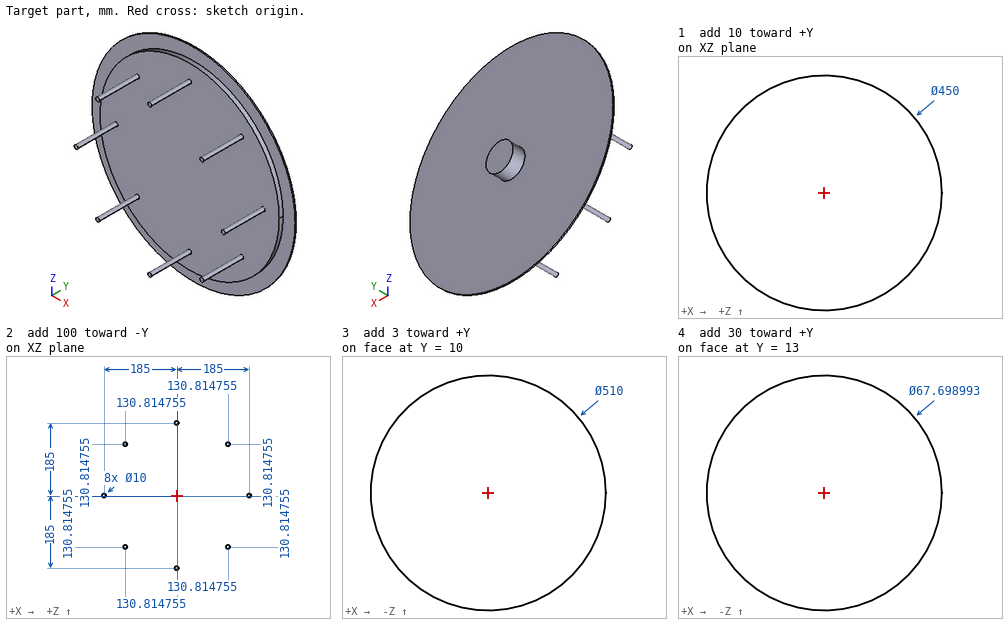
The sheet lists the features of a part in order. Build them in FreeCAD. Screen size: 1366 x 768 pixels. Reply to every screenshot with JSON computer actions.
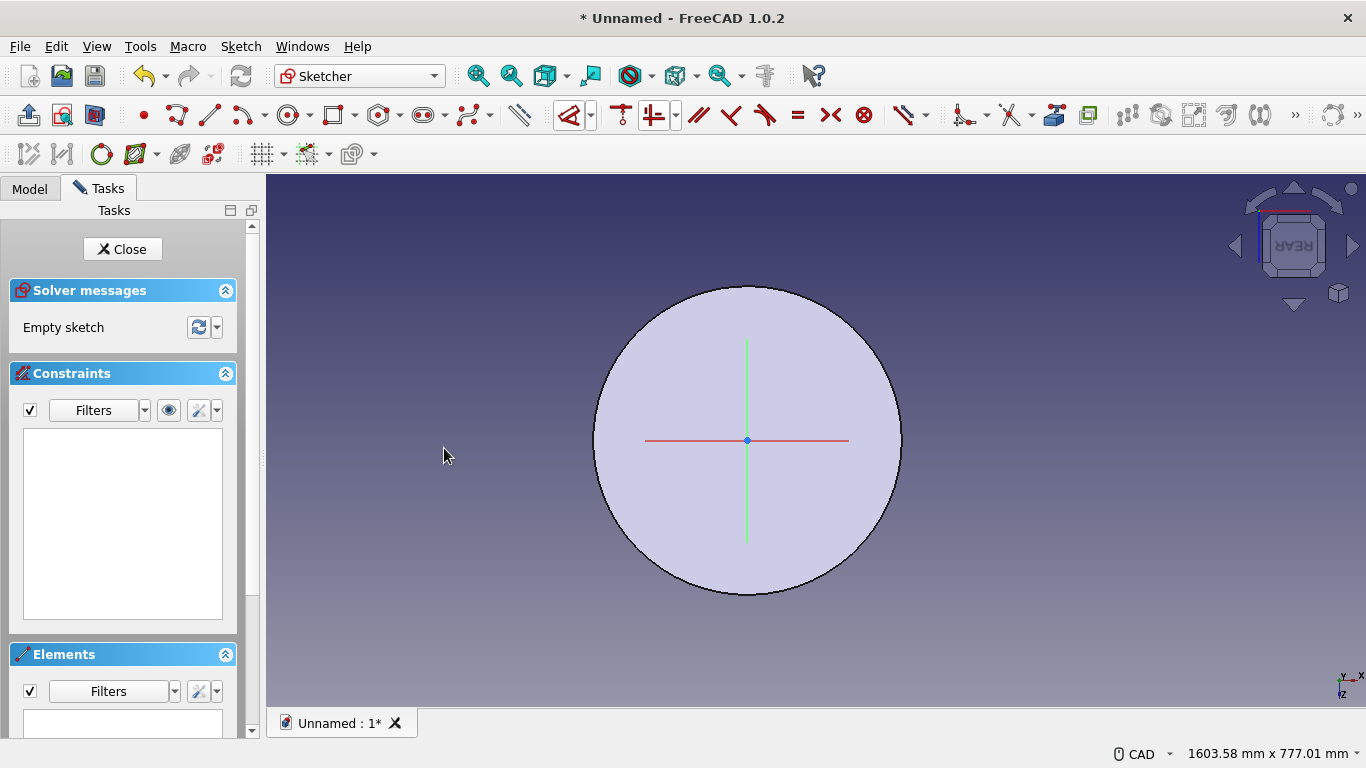
{"action": "left_click", "coordinate": [288, 116]}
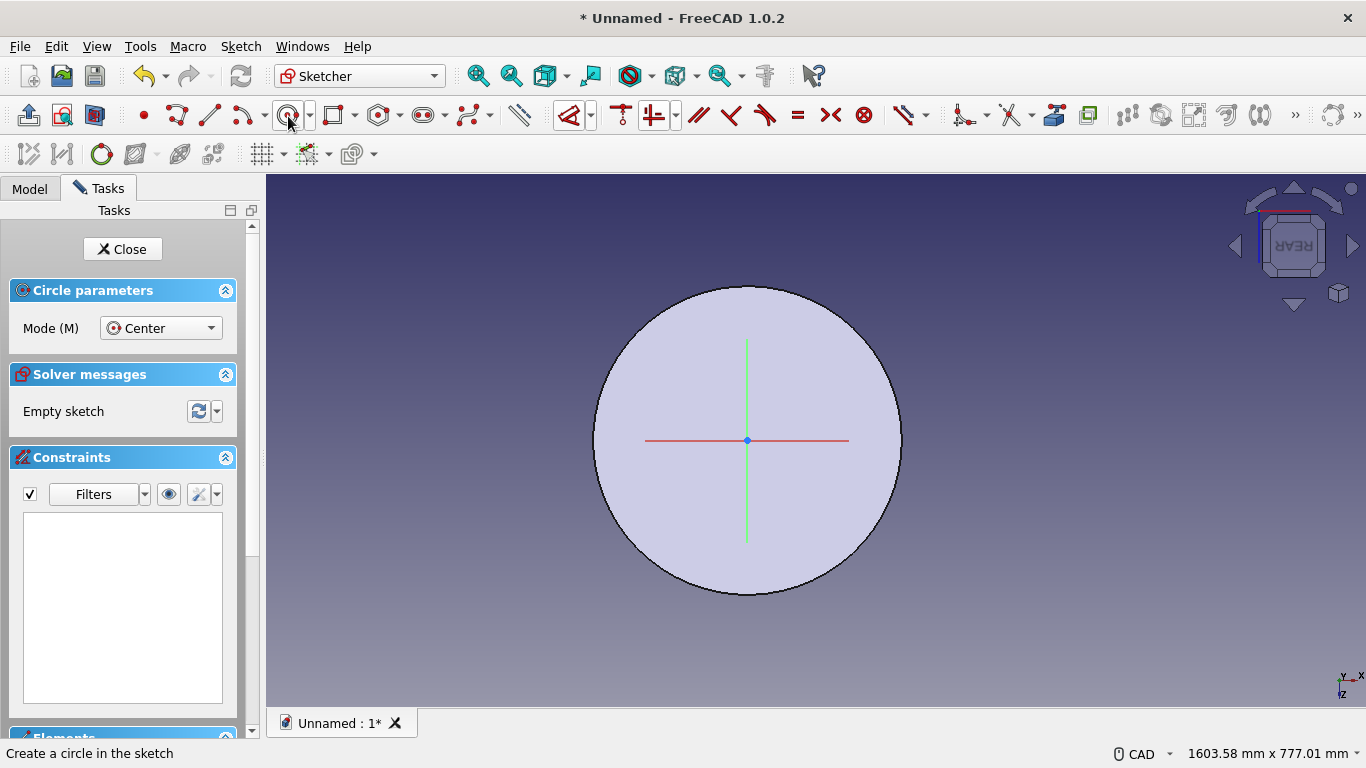
{"action": "left_click", "coordinate": [747, 441]}
{"action": "left_click", "coordinate": [871, 317]}
{"action": "key", "text": "Escape"}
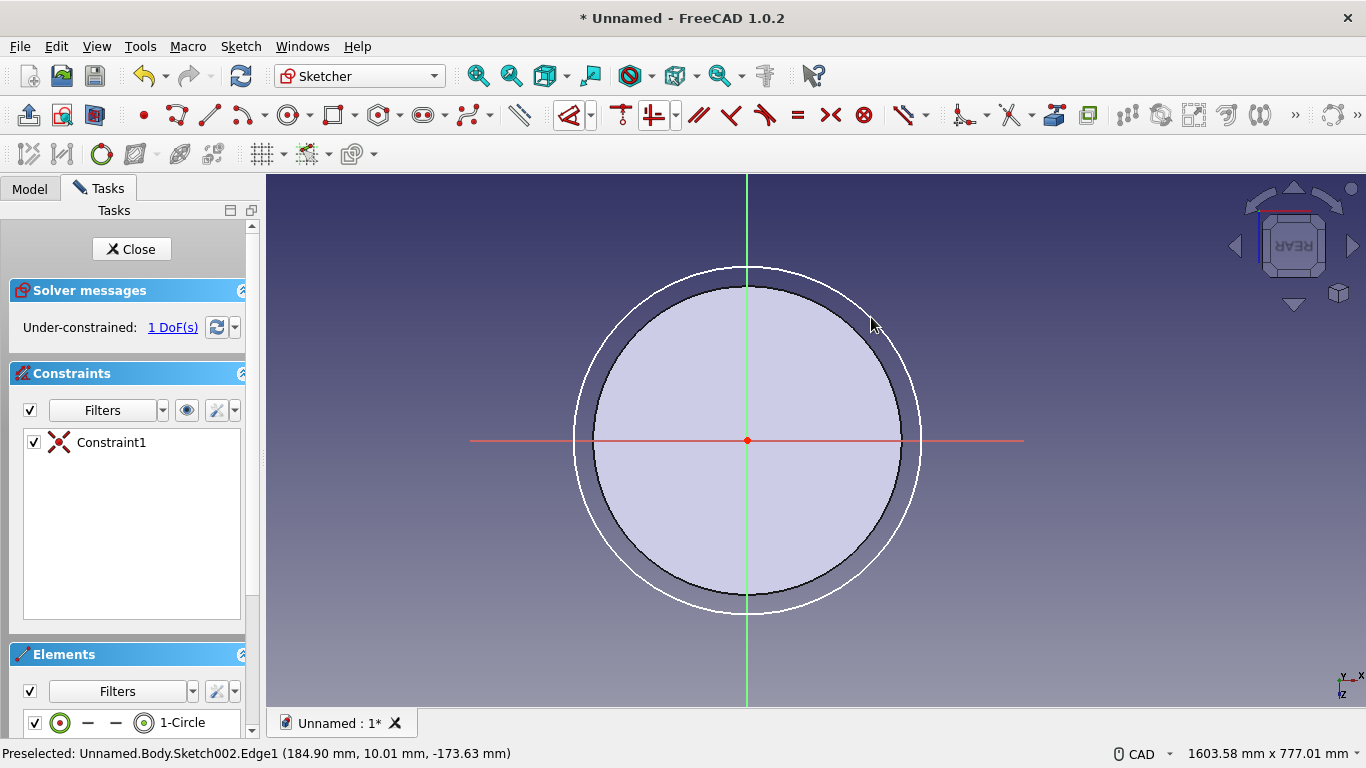
{"action": "left_click", "coordinate": [870, 317]}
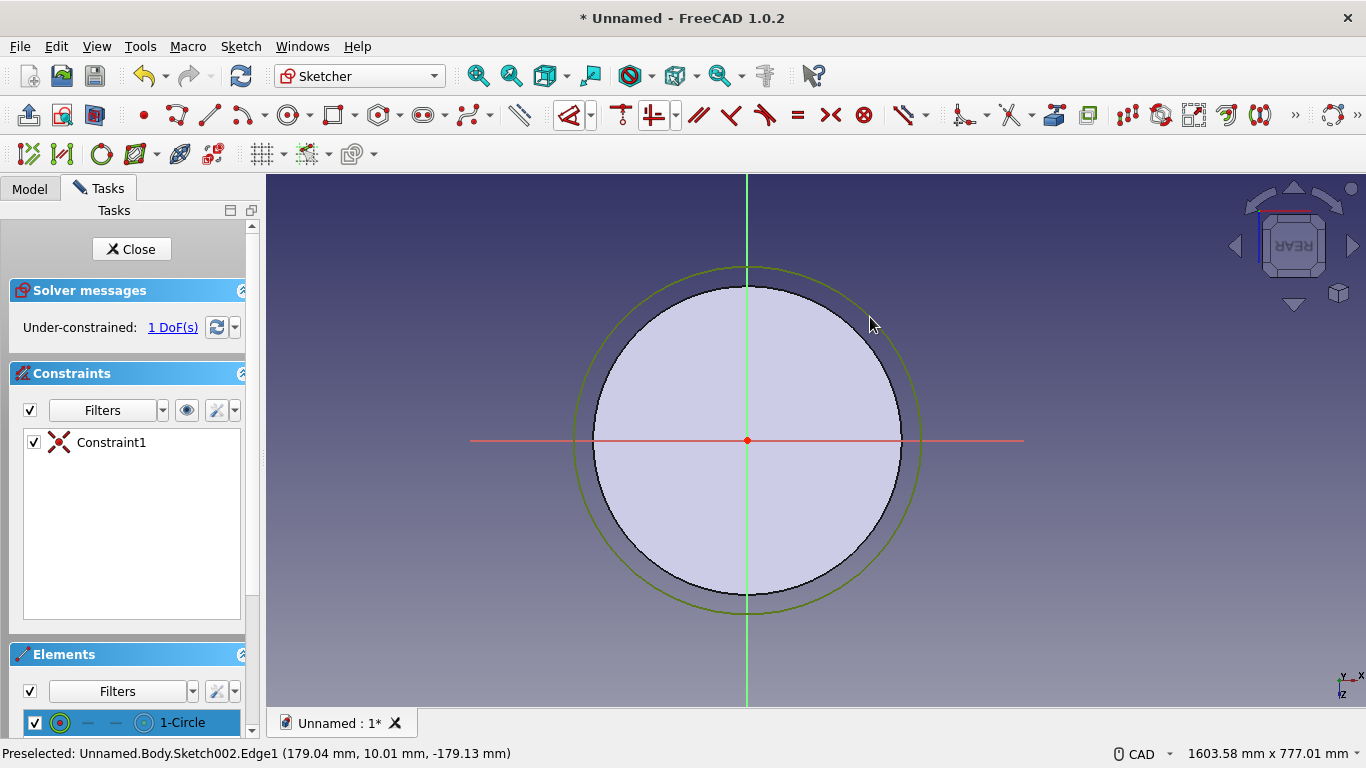
{"action": "key", "text": "k o"}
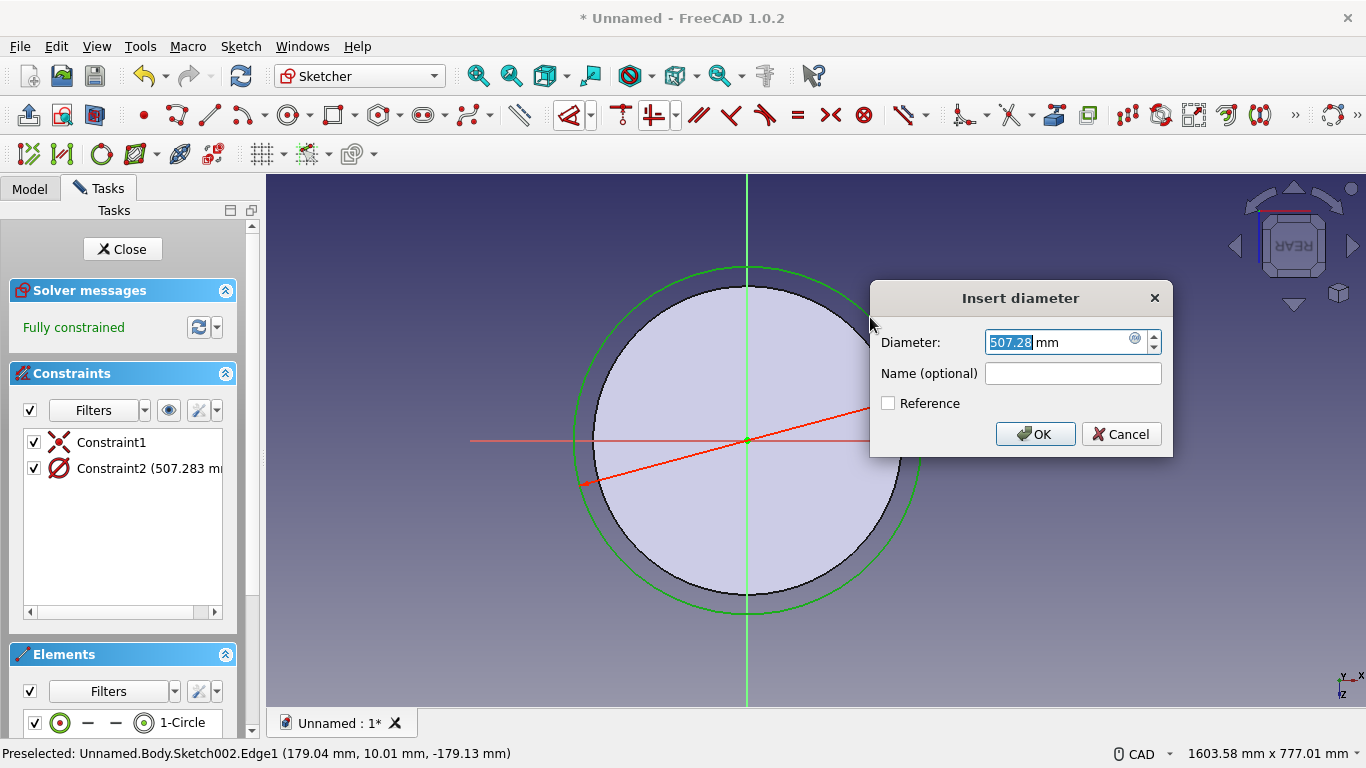
{"action": "type", "text": "510"}
{"action": "key", "text": "Return"}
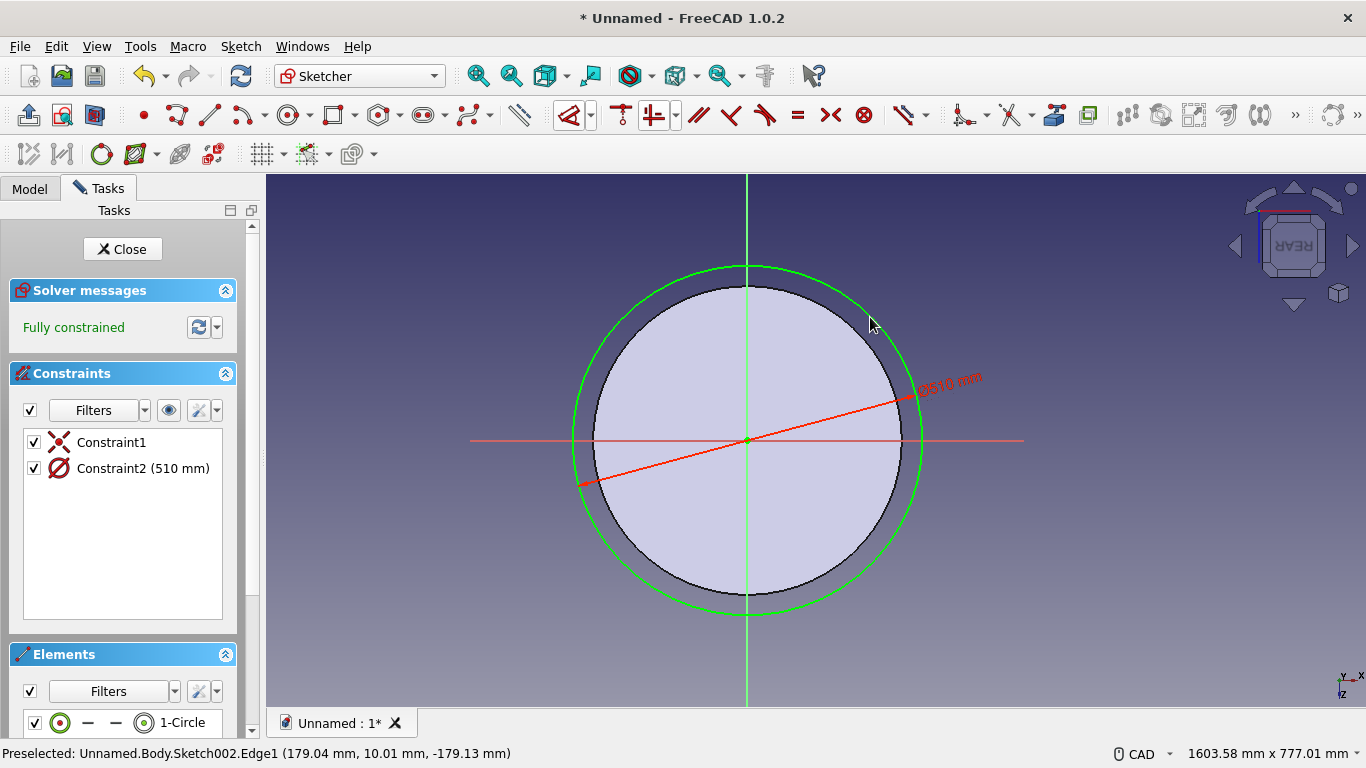
{"action": "left_click", "coordinate": [123, 249]}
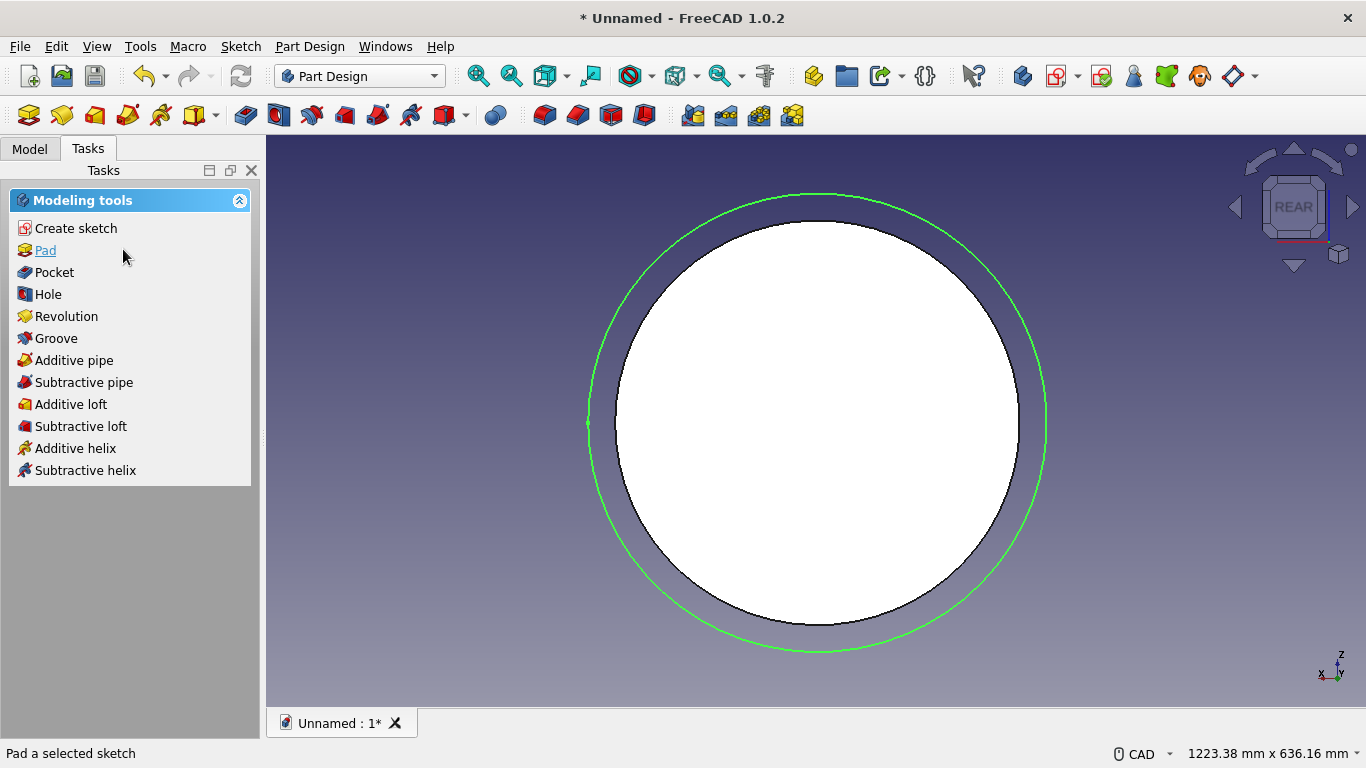
{"action": "left_click", "coordinate": [29, 116]}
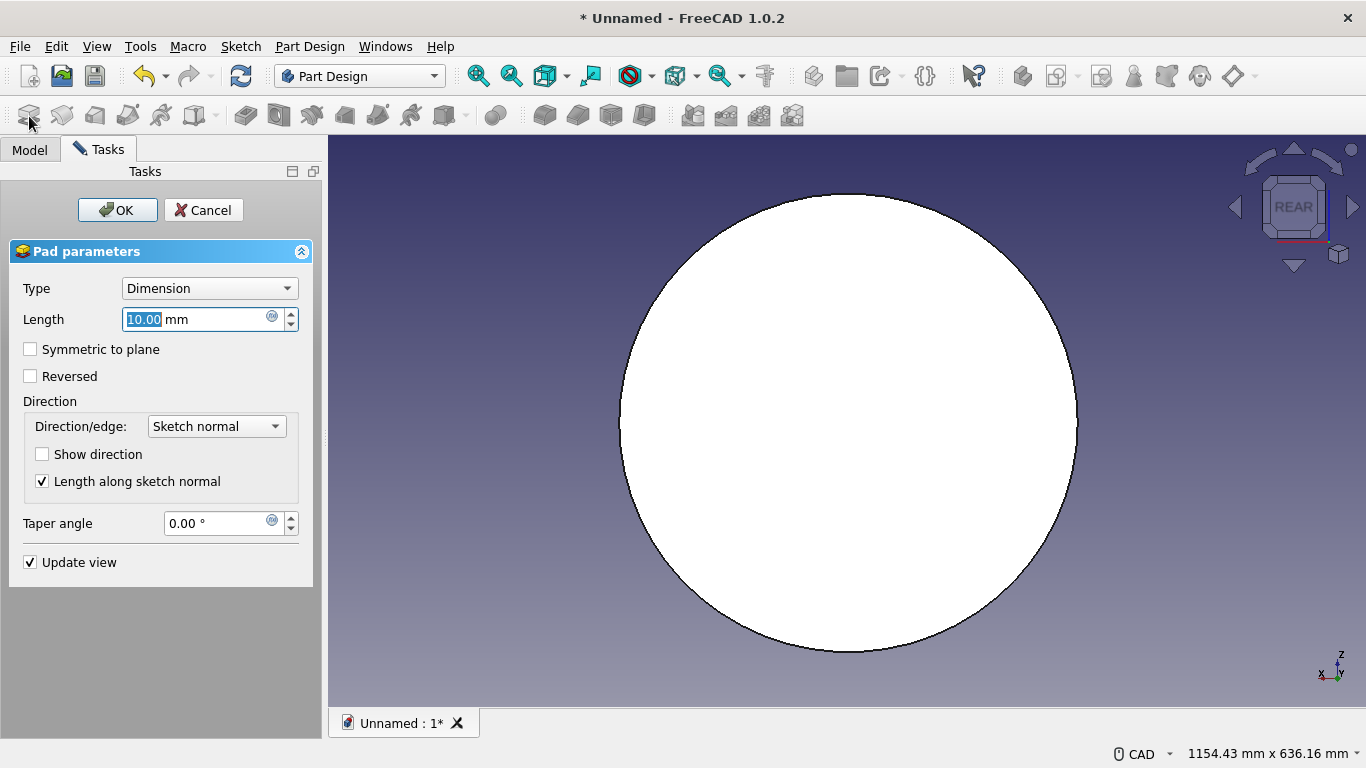
{"action": "type", "text": "3"}
{"action": "key", "text": "Tab"}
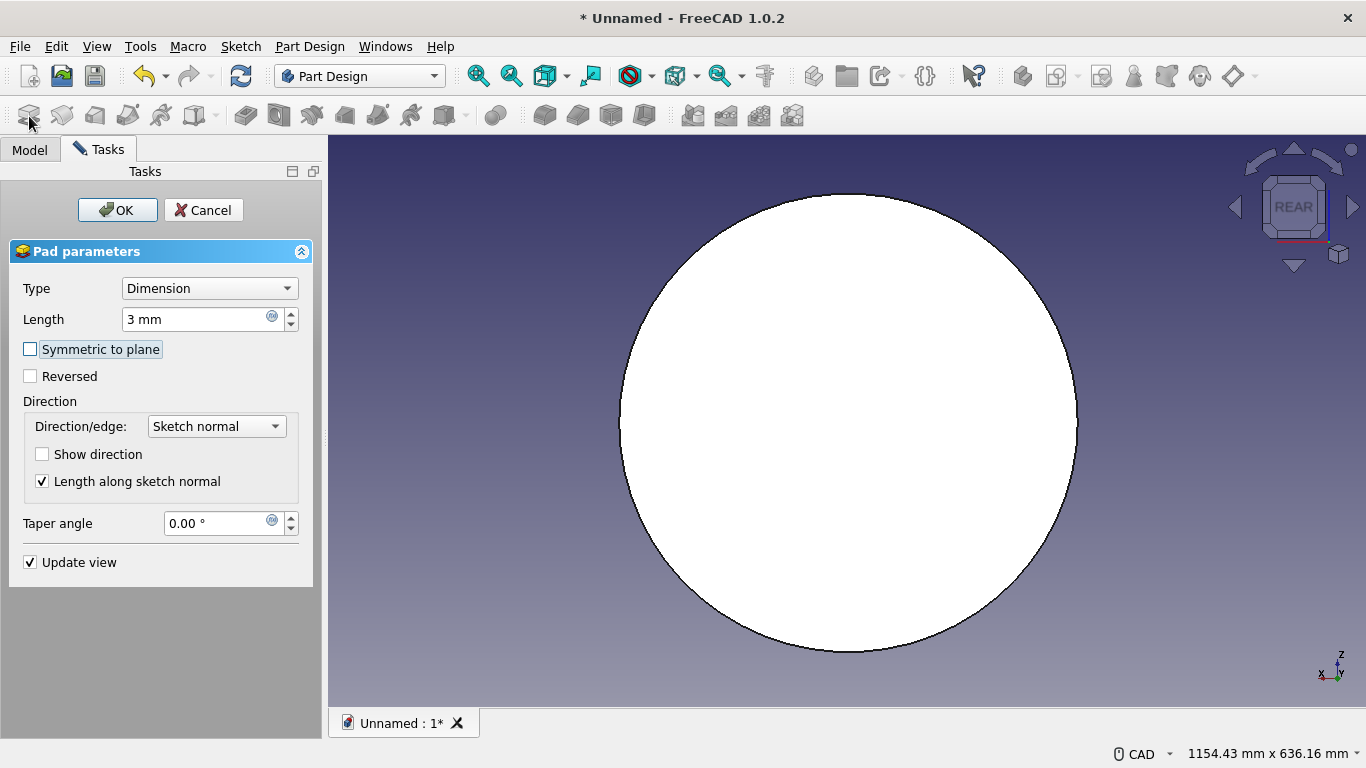
{"action": "left_click", "coordinate": [118, 210]}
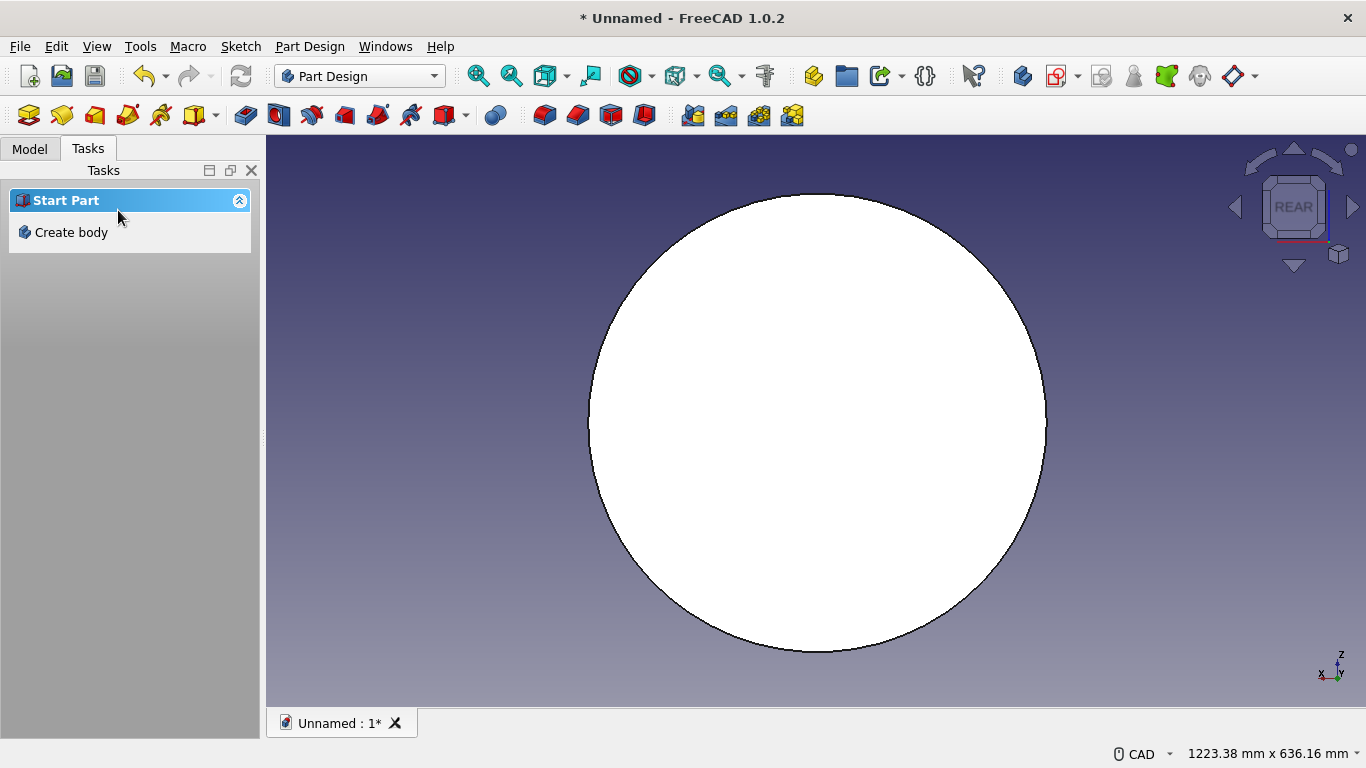
{"action": "left_click", "coordinate": [817, 422]}